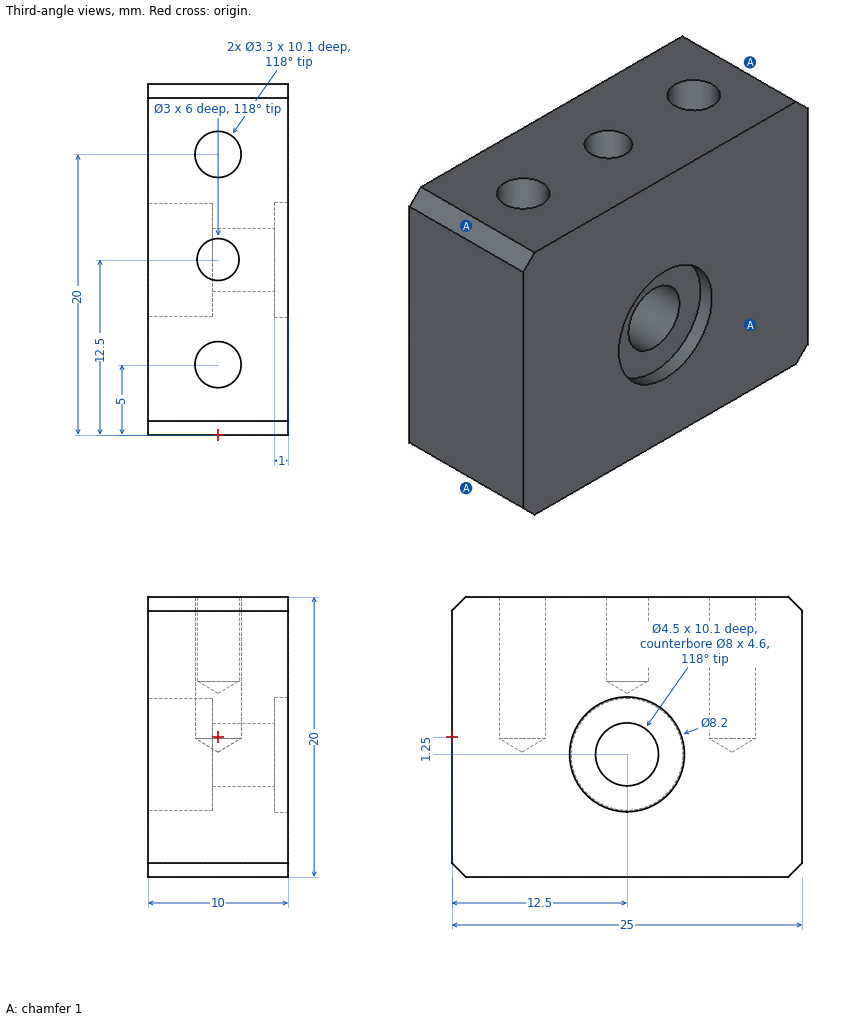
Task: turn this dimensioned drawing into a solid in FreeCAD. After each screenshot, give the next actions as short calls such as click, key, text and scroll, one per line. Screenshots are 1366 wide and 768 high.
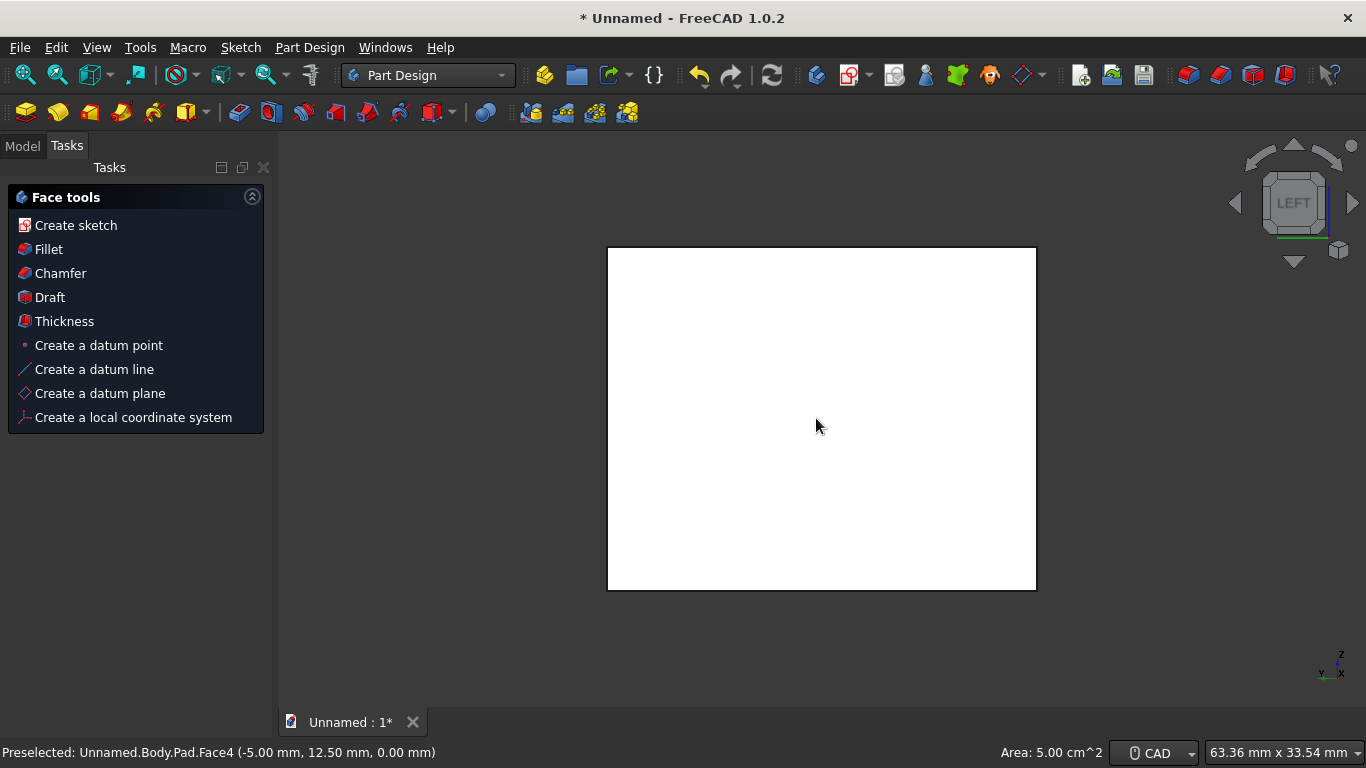
click(850, 76)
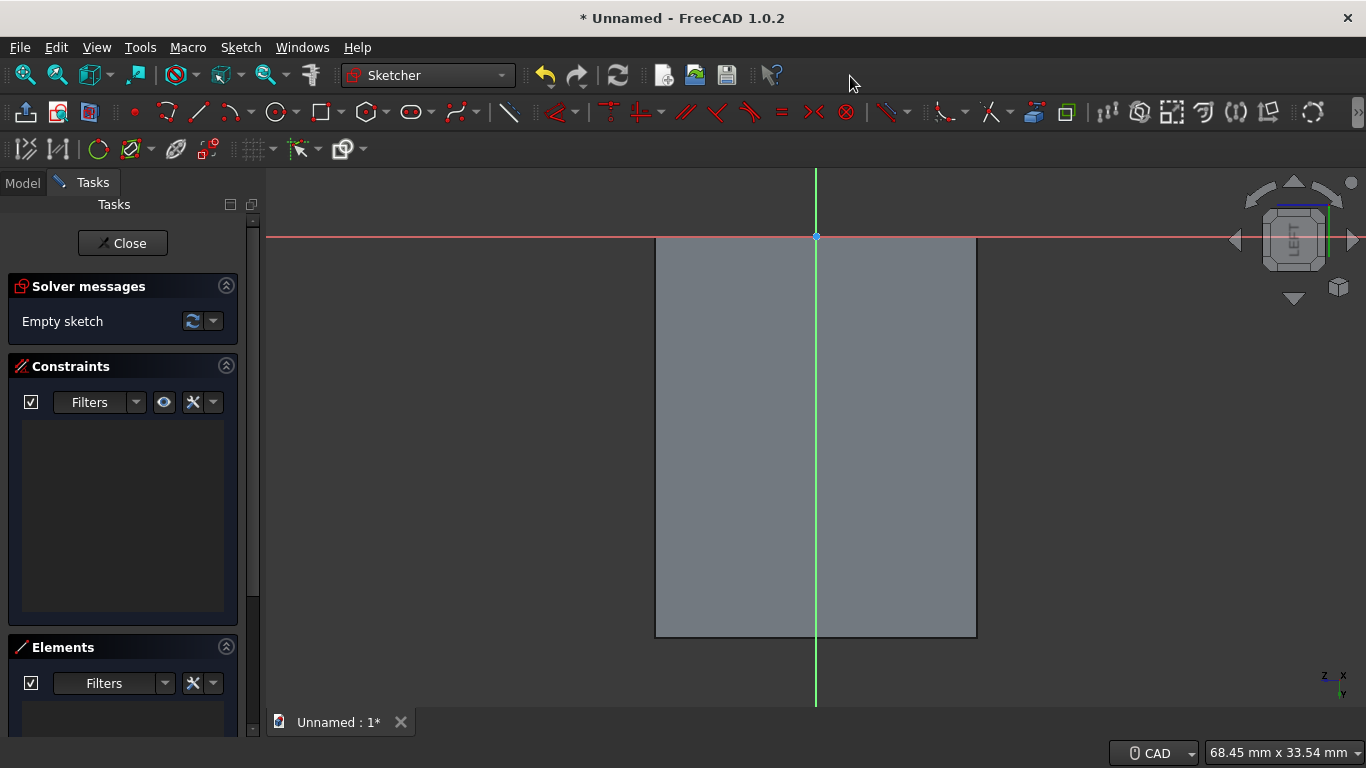
scroll(858, 437, up, 8)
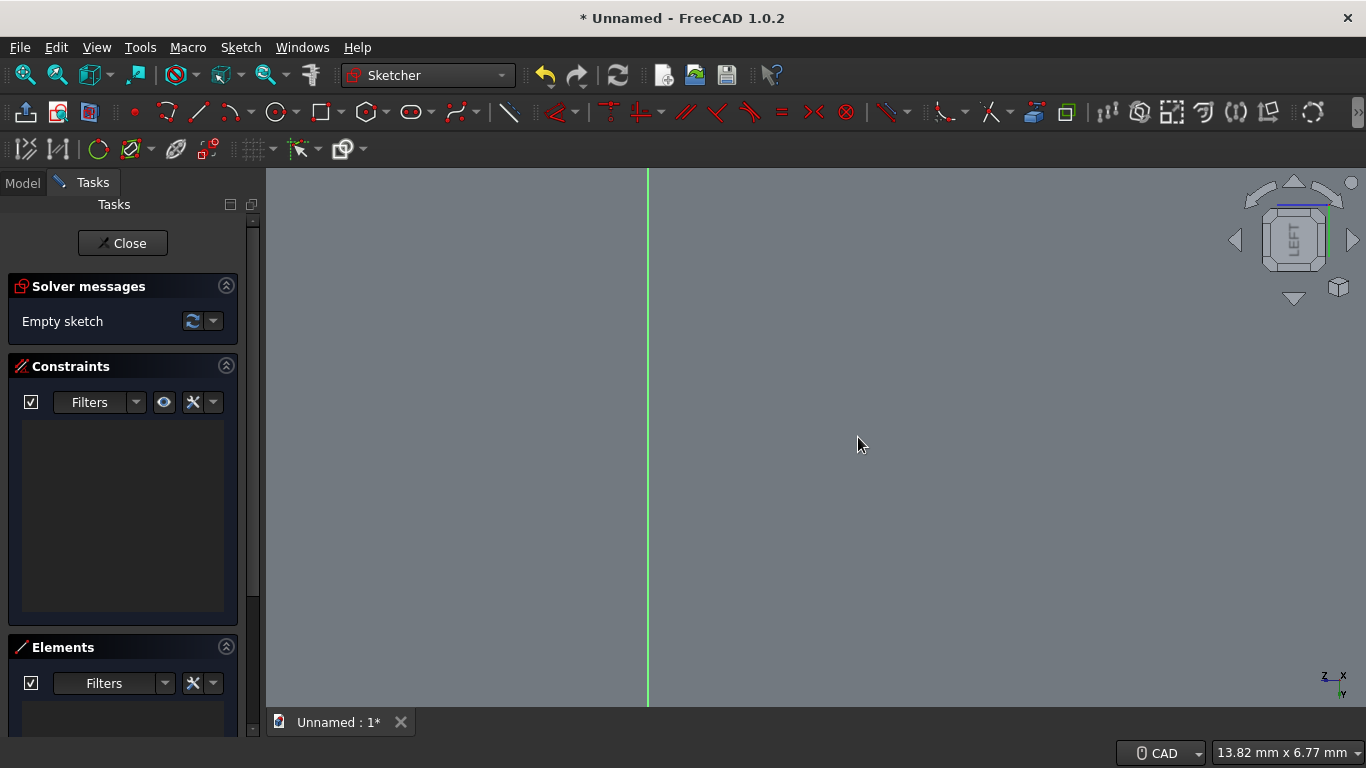
key(g)
key(c)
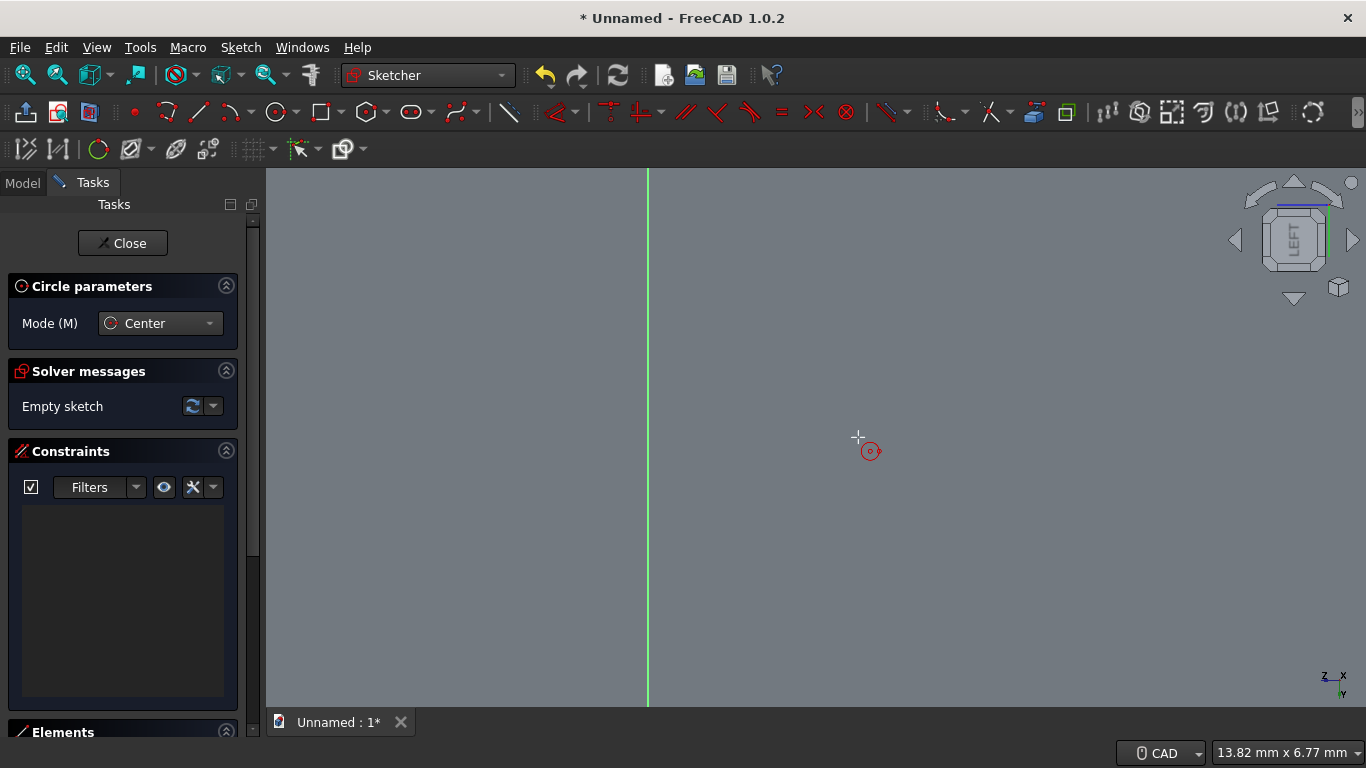
click(747, 437)
click(874, 311)
key(Escape)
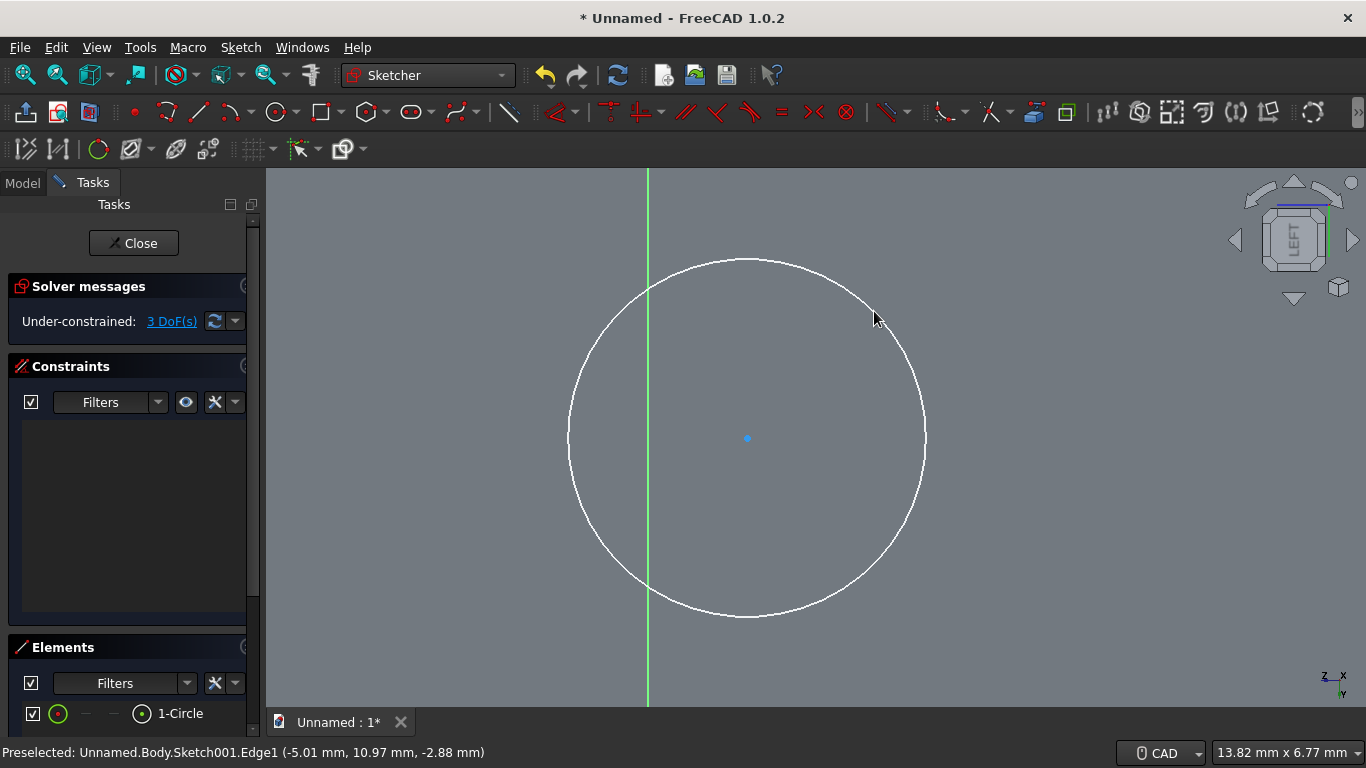
click(556, 112)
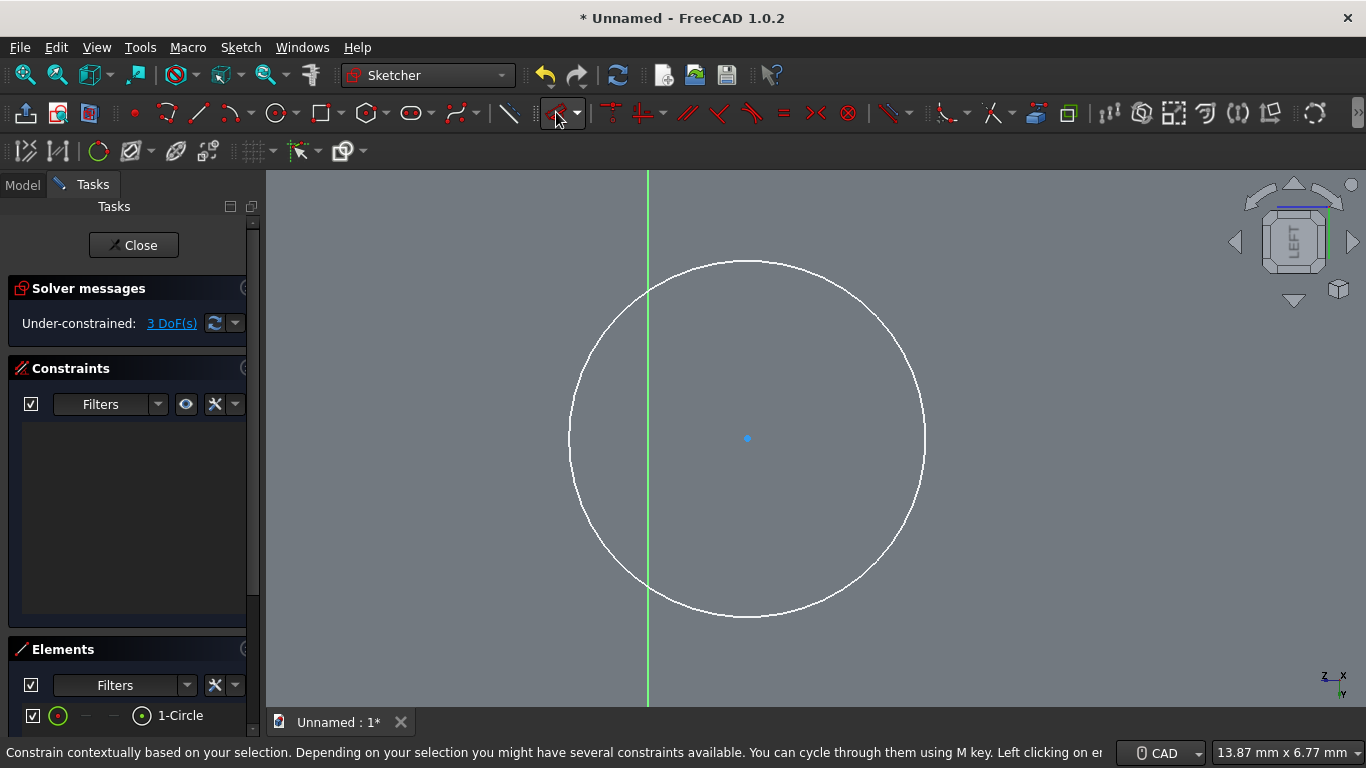
click(873, 313)
click(896, 290)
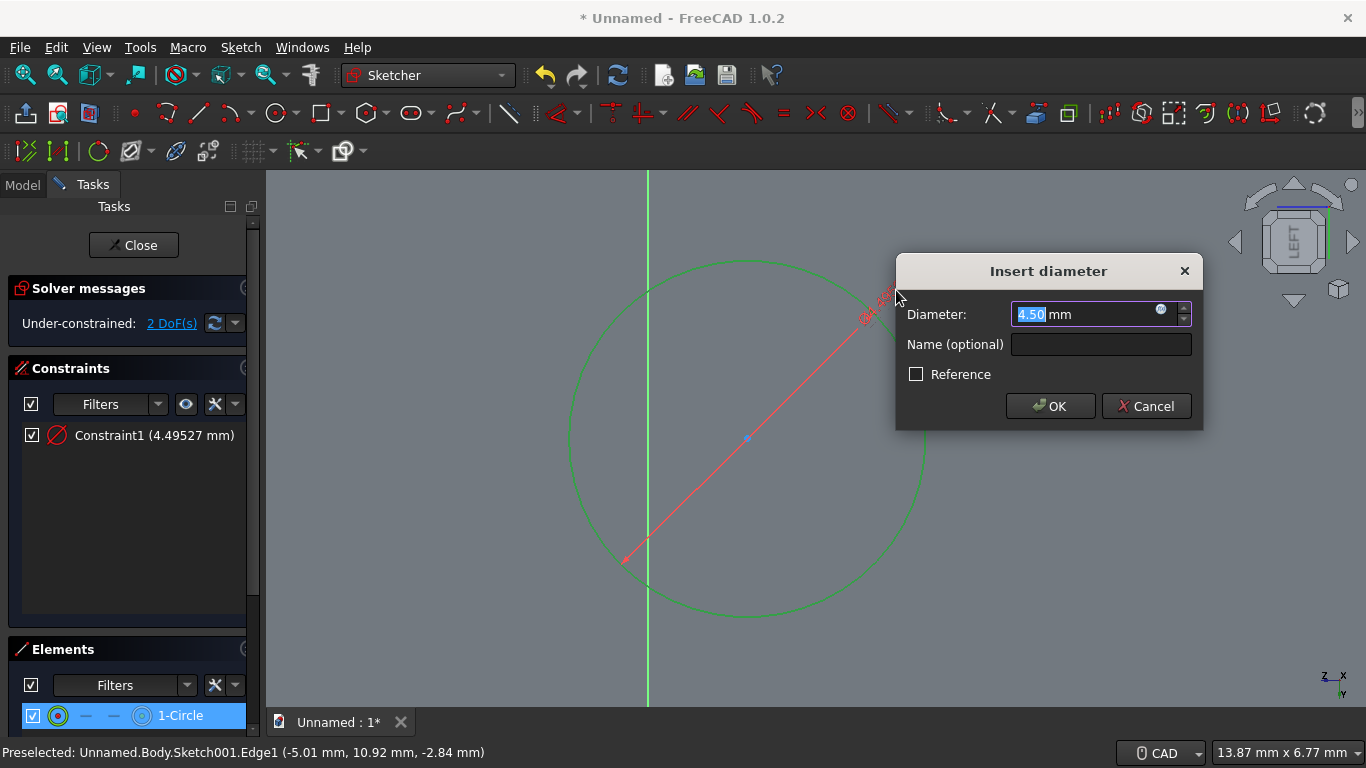
text(4.5)
key(Return)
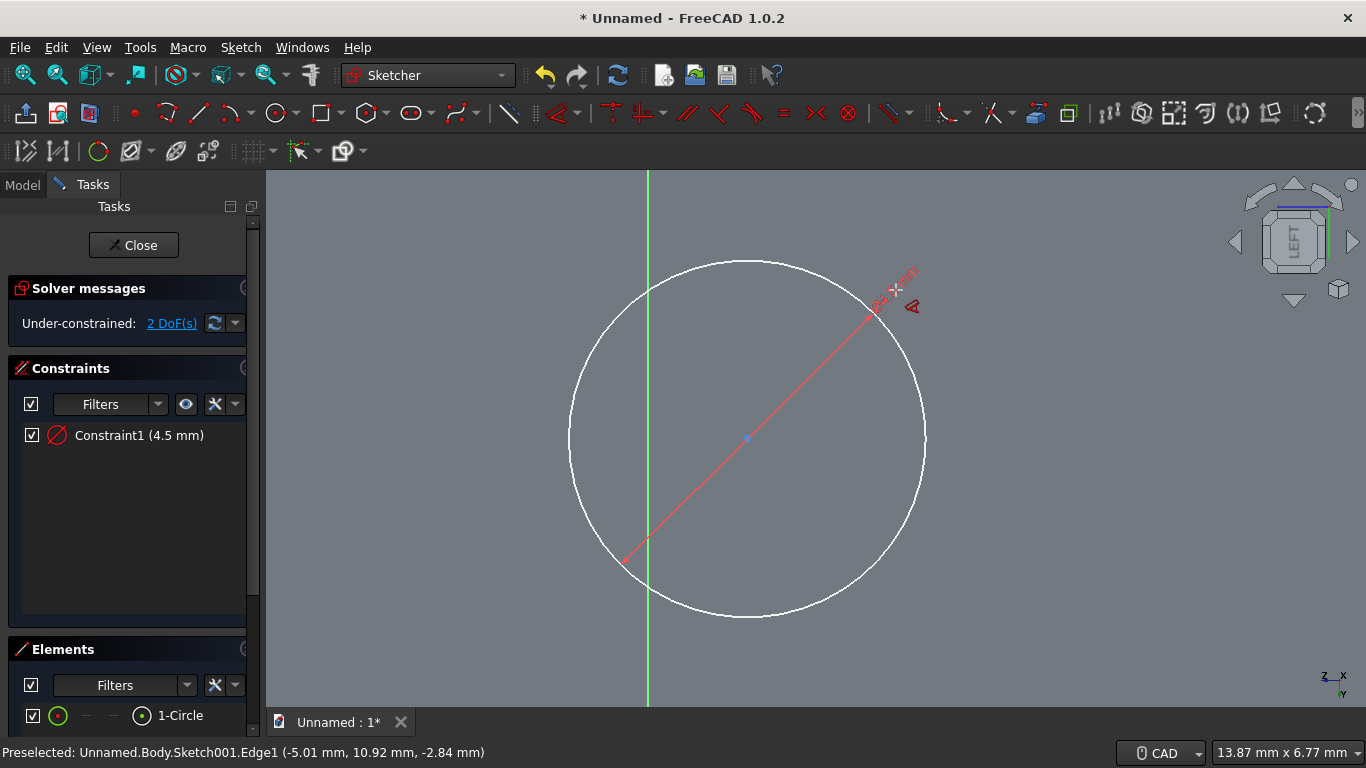
click(747, 439)
click(698, 473)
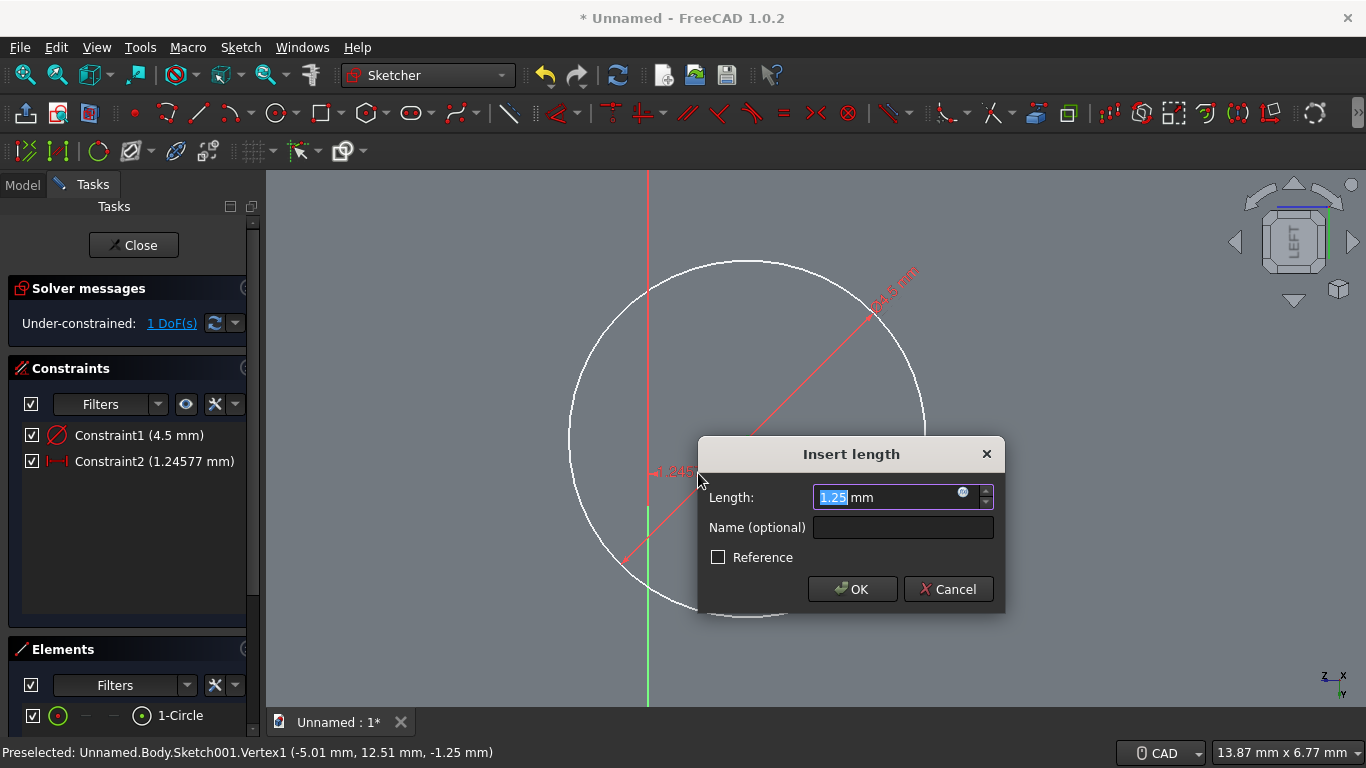
text(1.25)
key(Return)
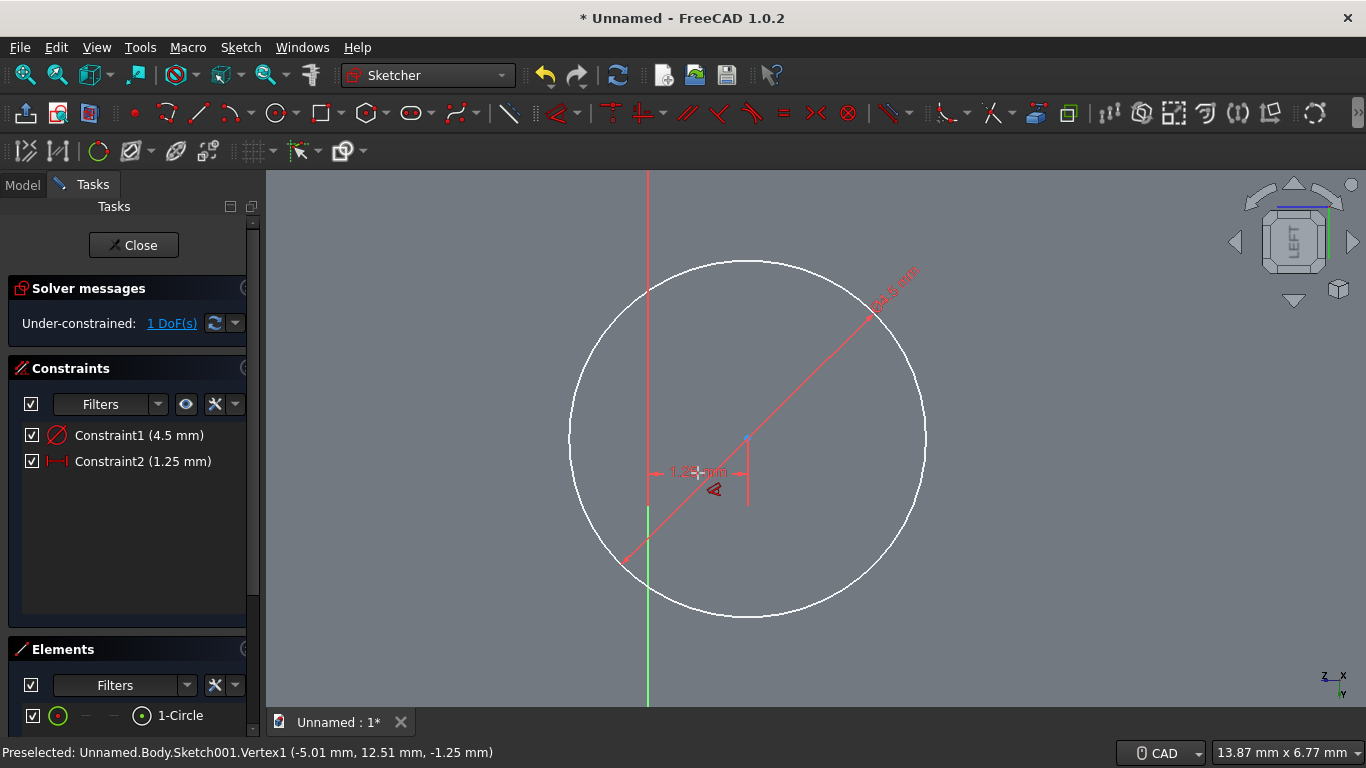
click(748, 439)
click(614, 263)